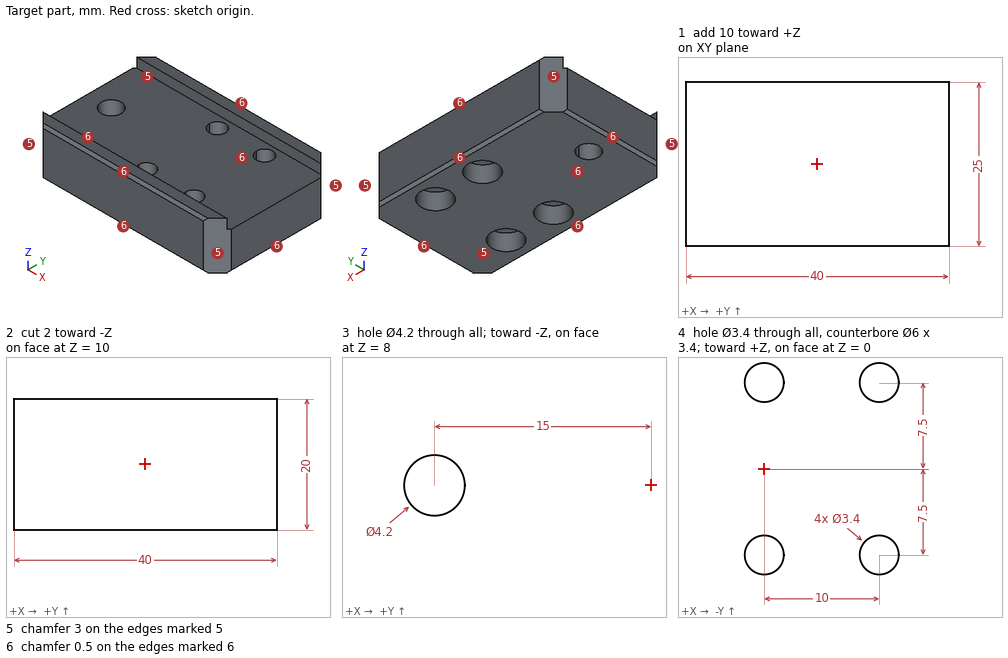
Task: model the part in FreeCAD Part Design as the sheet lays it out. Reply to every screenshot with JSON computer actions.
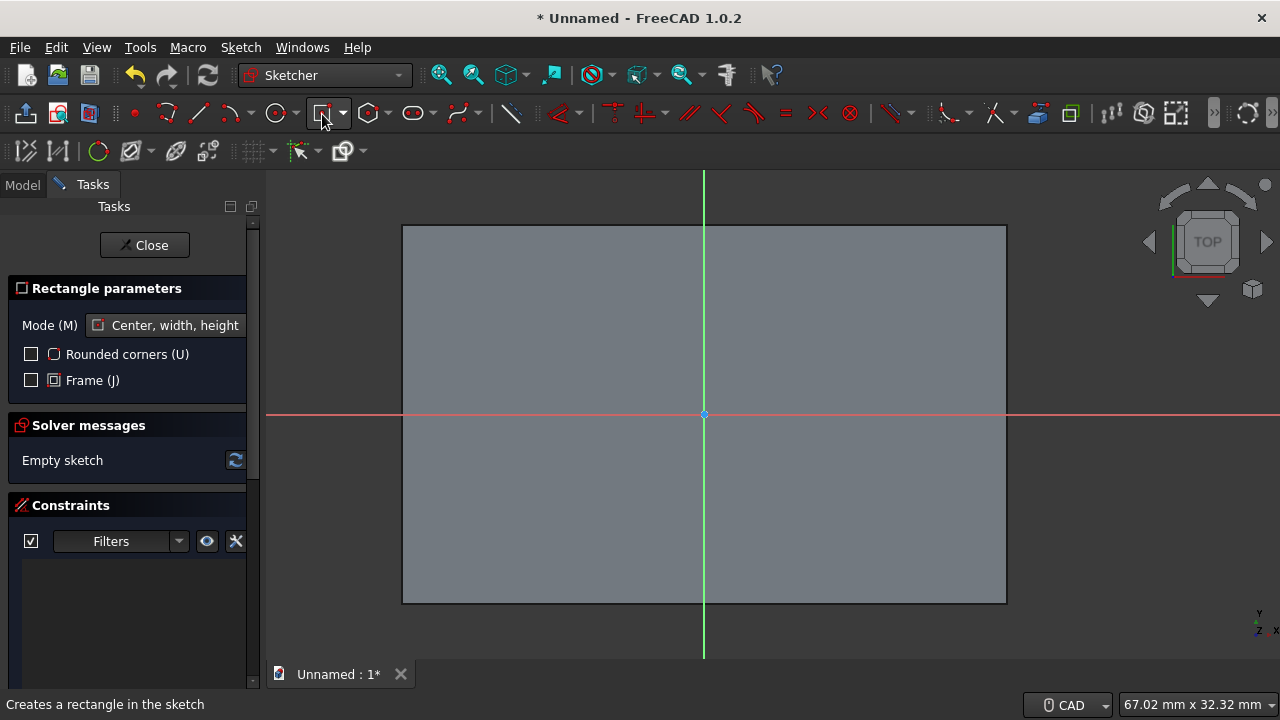
{"action": "left_click", "coordinate": [704, 414]}
{"action": "left_click", "coordinate": [1007, 263]}
{"action": "key", "text": "Escape"}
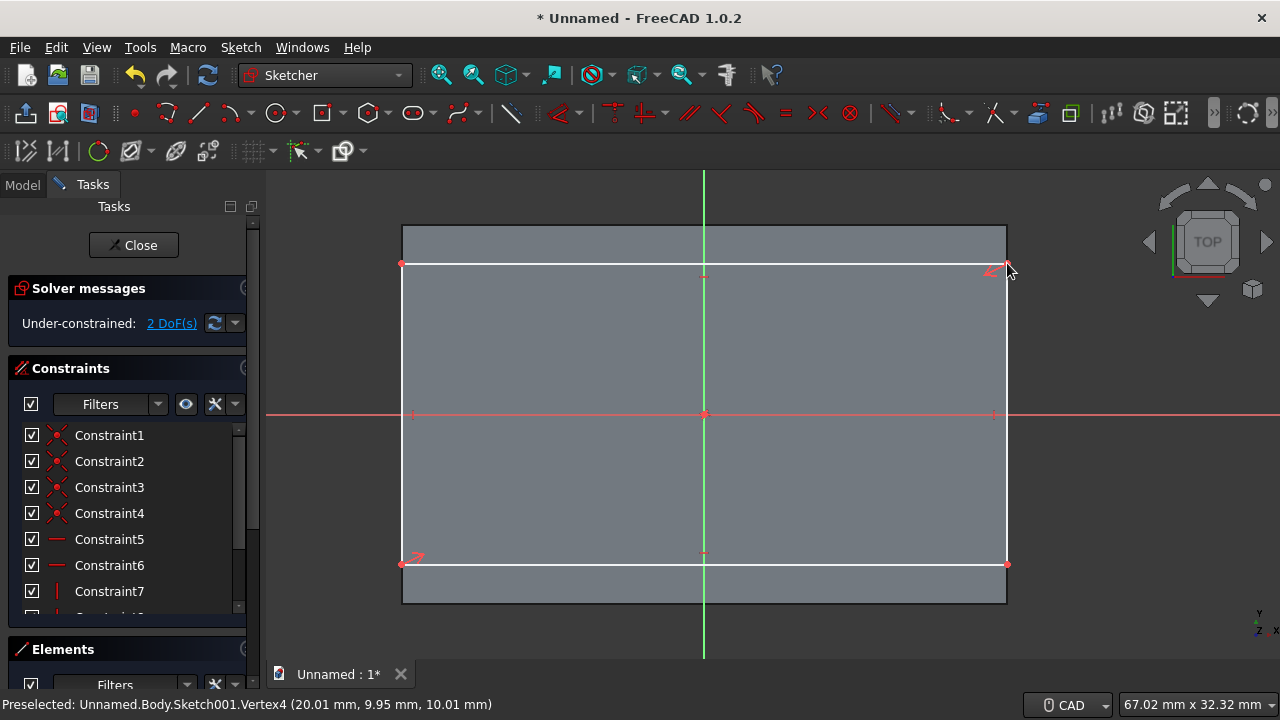
{"action": "left_click", "coordinate": [558, 114]}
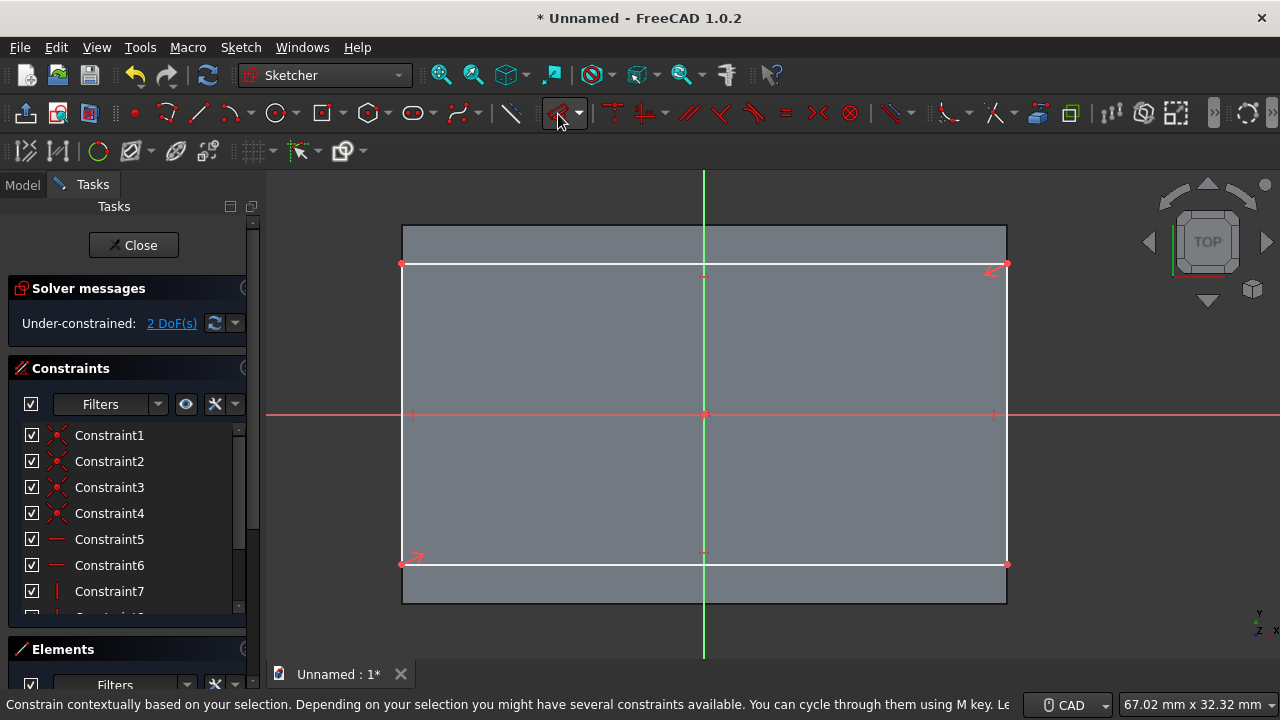
{"action": "left_click", "coordinate": [583, 565]}
{"action": "left_click", "coordinate": [565, 599]}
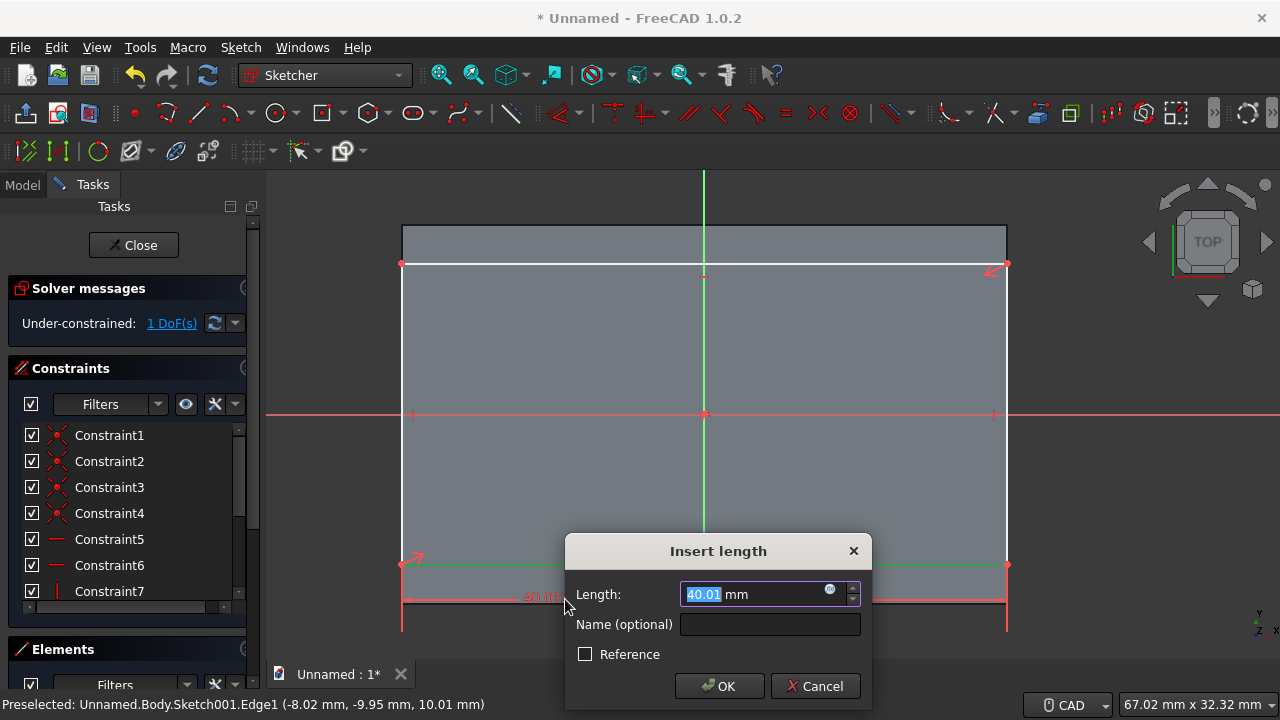
{"action": "type", "text": "40"}
{"action": "key", "text": "Return"}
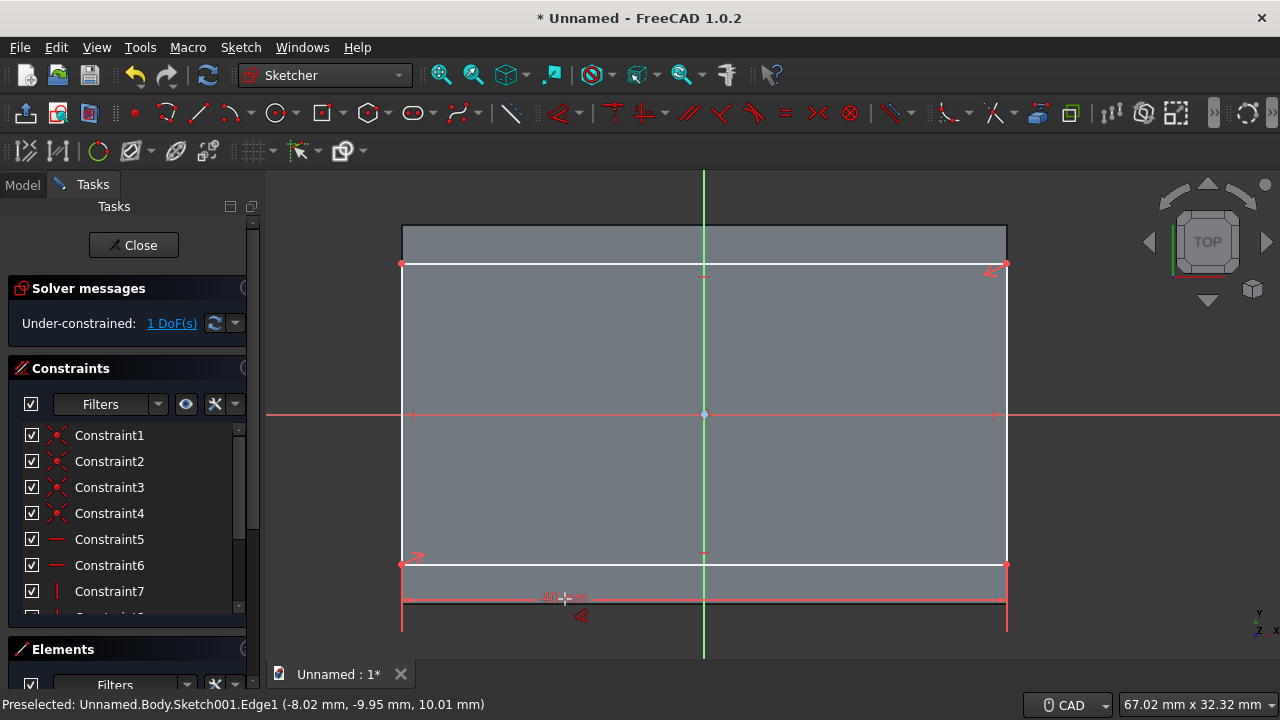
{"action": "left_click", "coordinate": [1007, 475]}
{"action": "left_click", "coordinate": [1041, 345]}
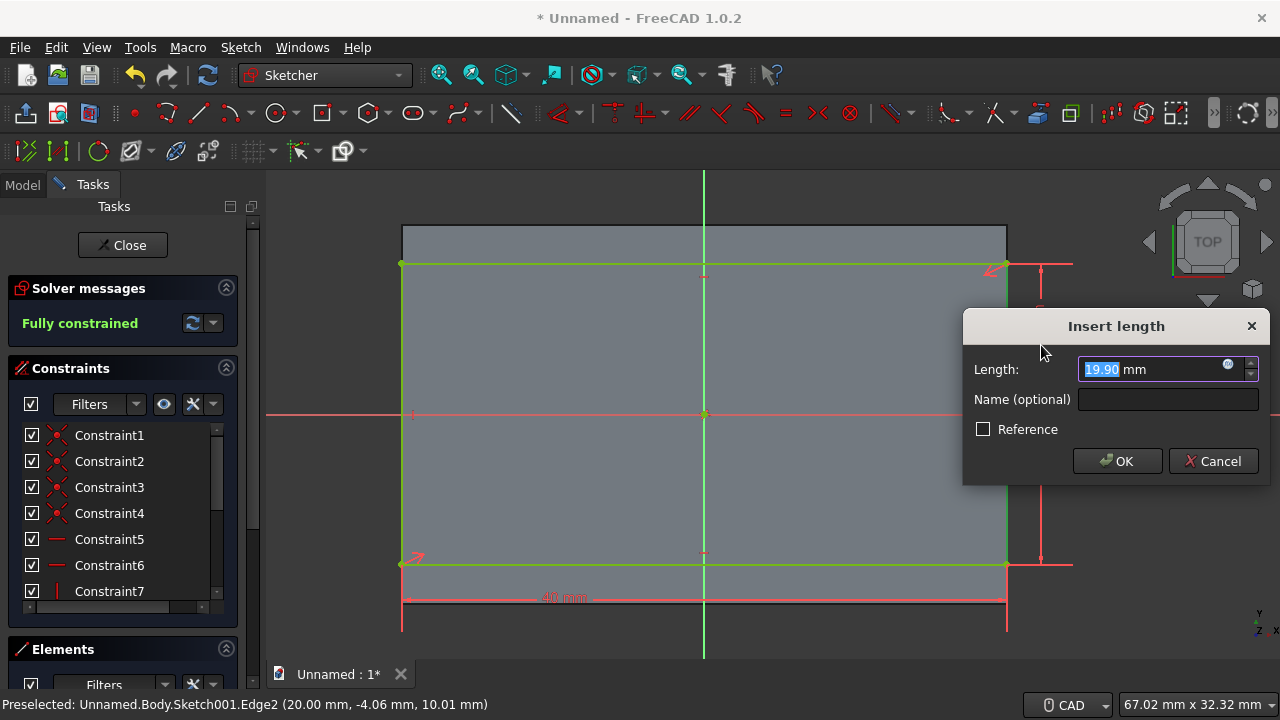
{"action": "type", "text": "20"}
{"action": "key", "text": "Return"}
{"action": "key", "text": "Escape"}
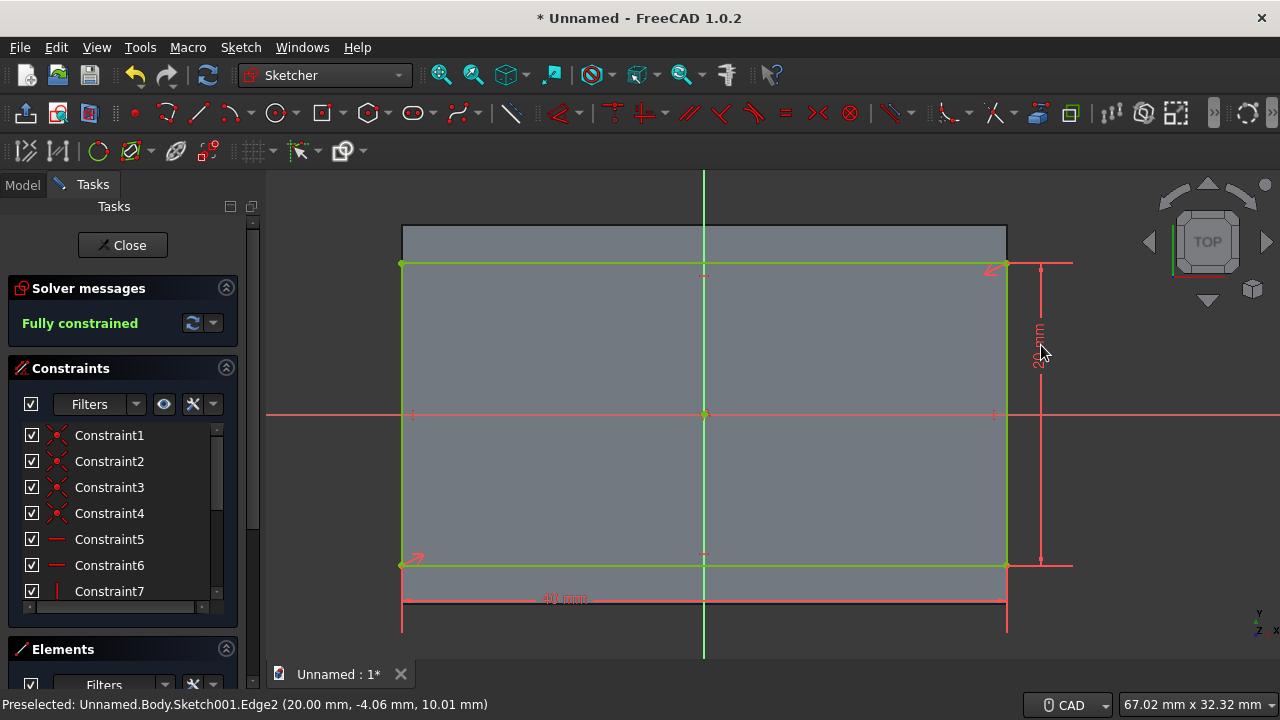
{"action": "left_click", "coordinate": [123, 245]}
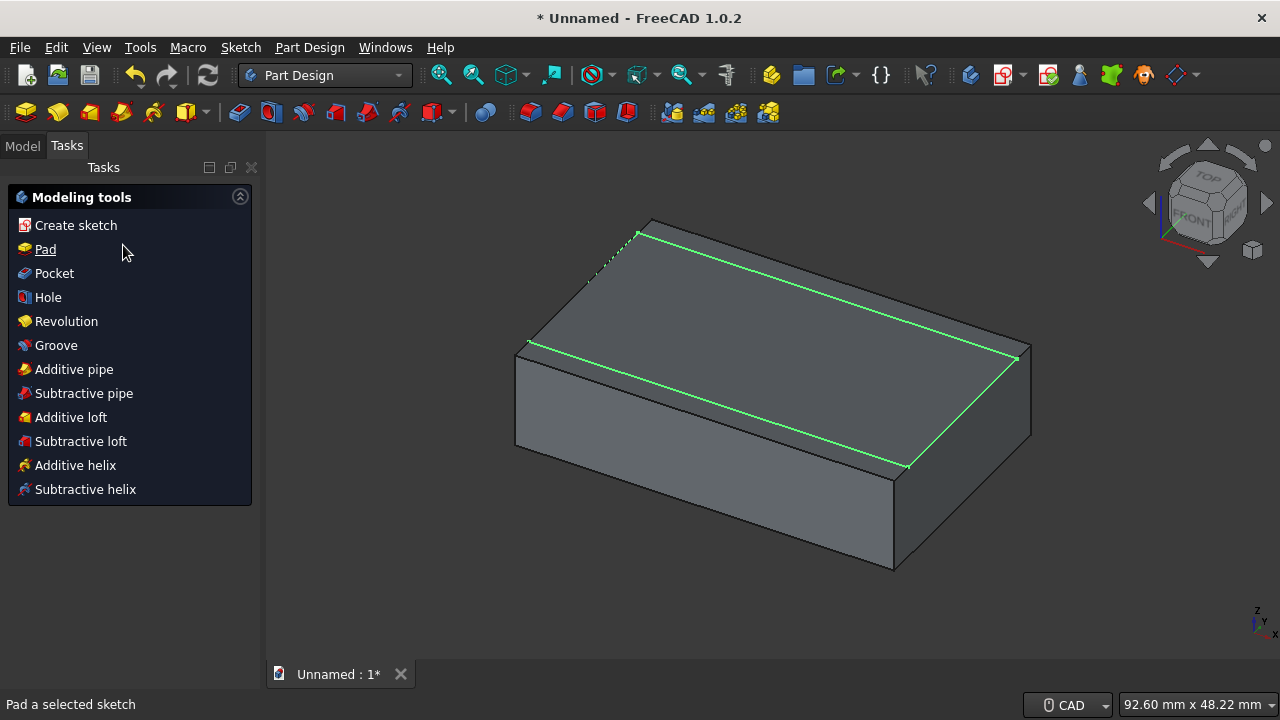
{"action": "left_click", "coordinate": [240, 112]}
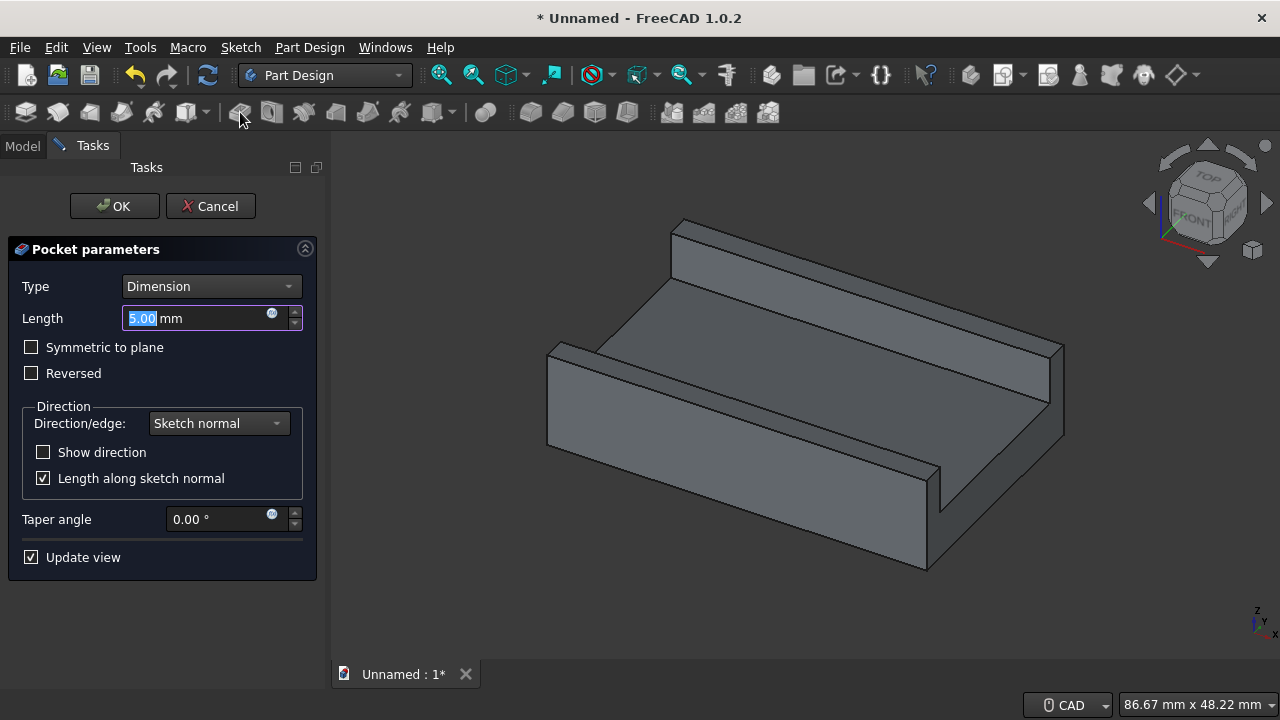
{"action": "type", "text": "2"}
{"action": "key", "text": "Tab"}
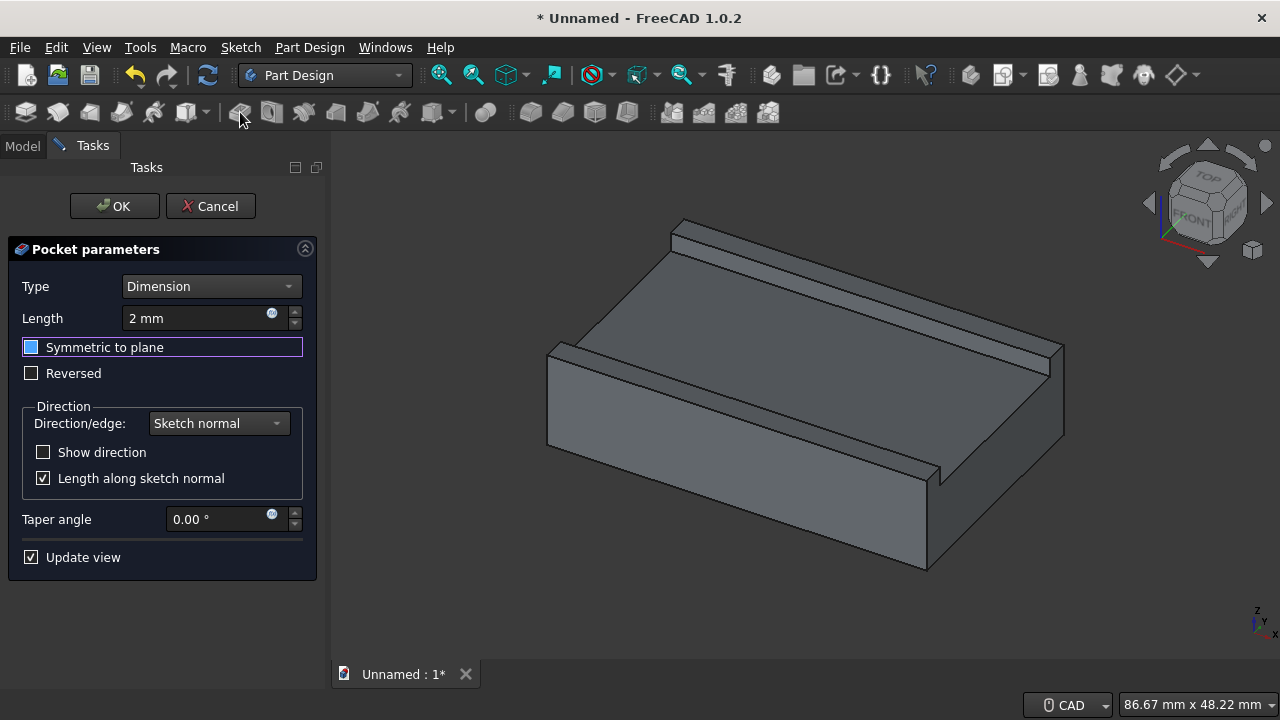
{"action": "left_click", "coordinate": [115, 206]}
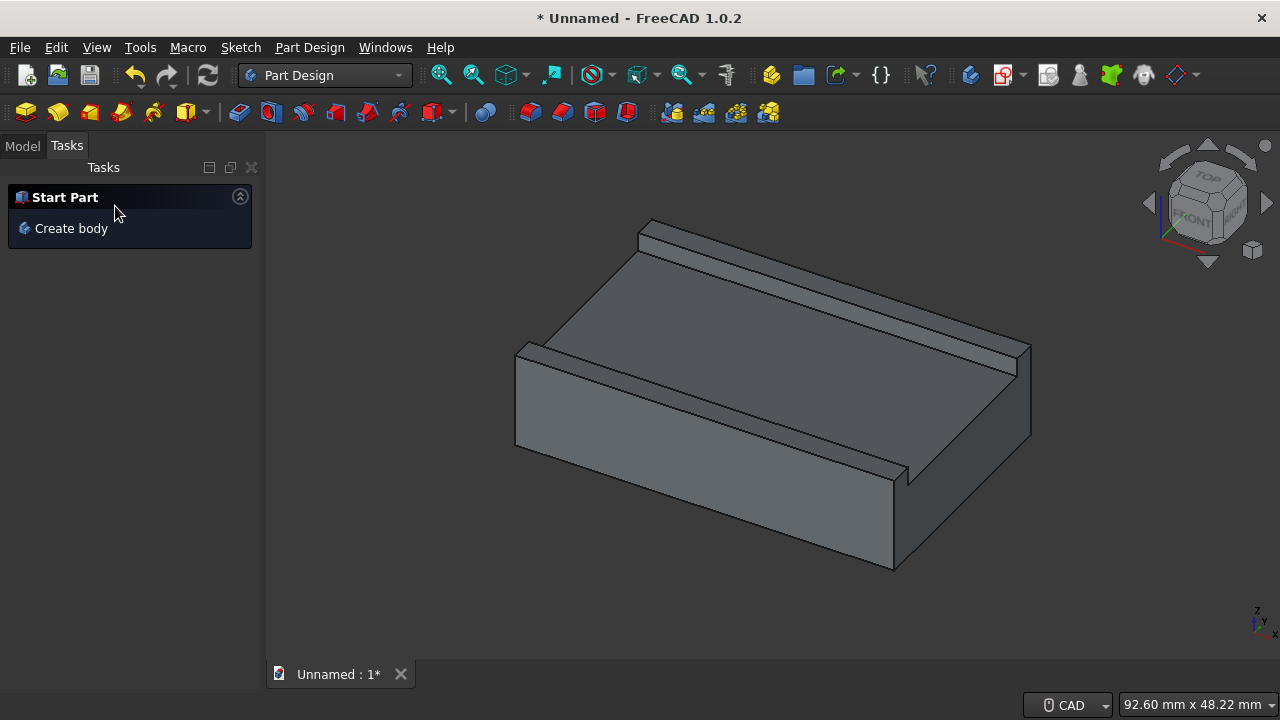
{"action": "left_click", "coordinate": [827, 385]}